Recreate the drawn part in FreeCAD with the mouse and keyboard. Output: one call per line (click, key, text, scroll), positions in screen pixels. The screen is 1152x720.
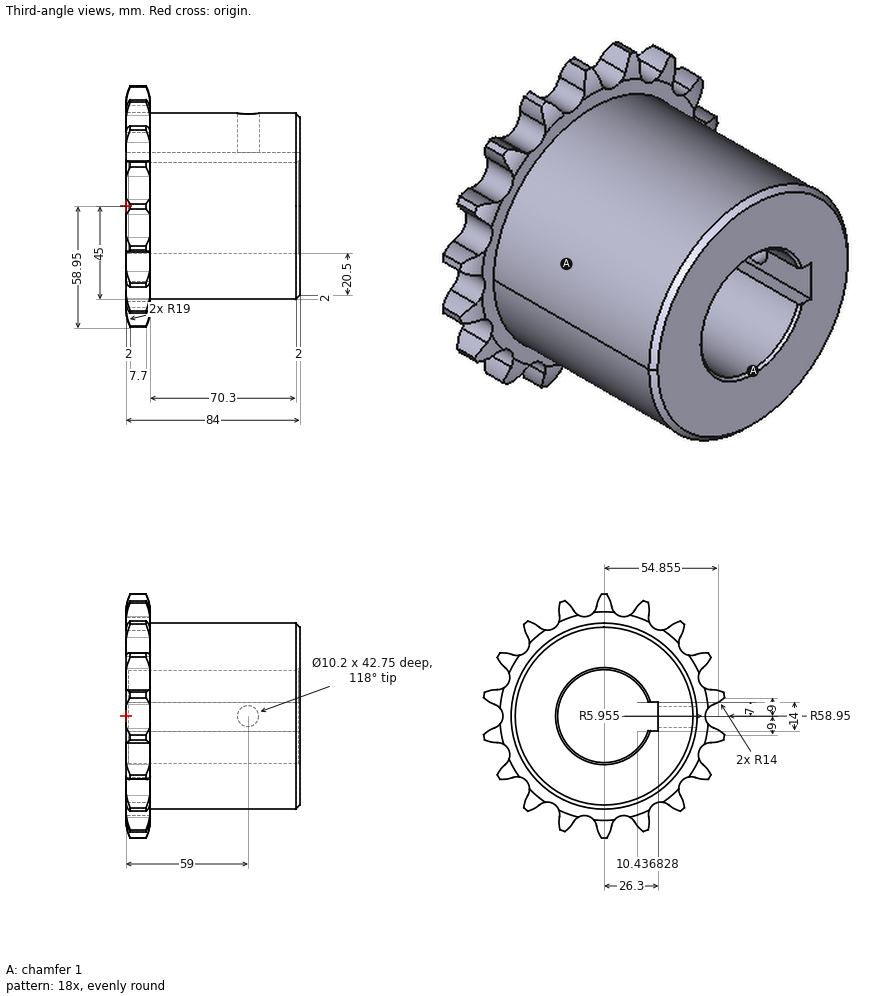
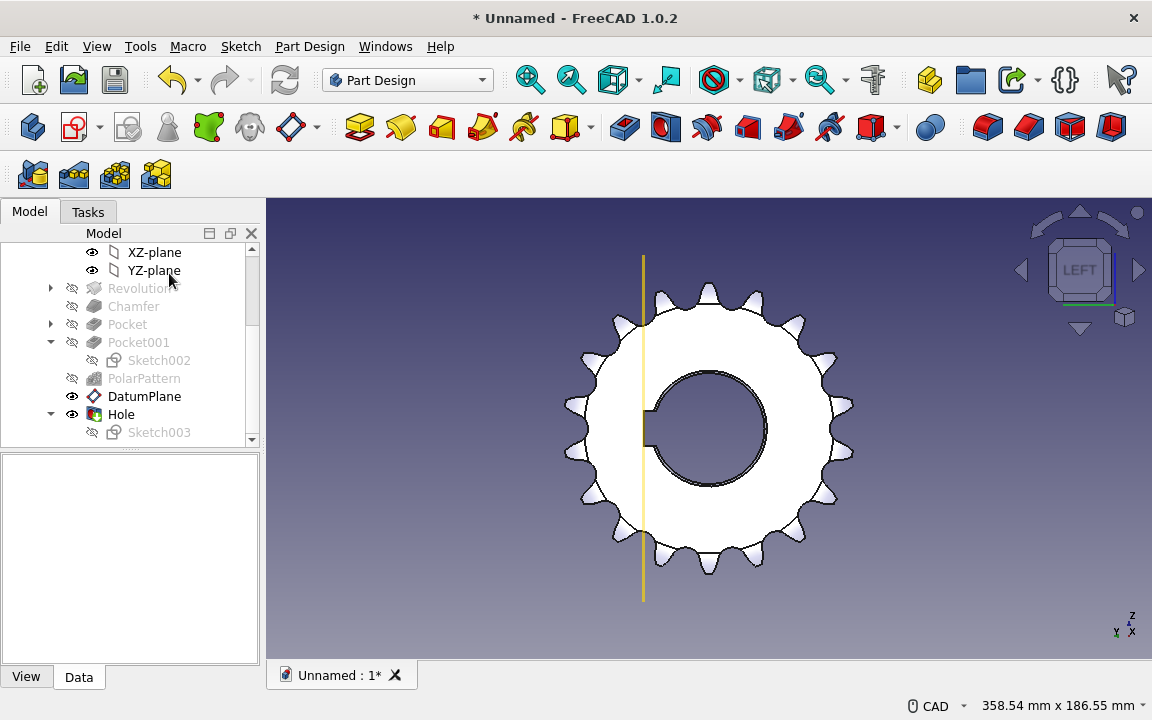
click(117, 396)
key(space)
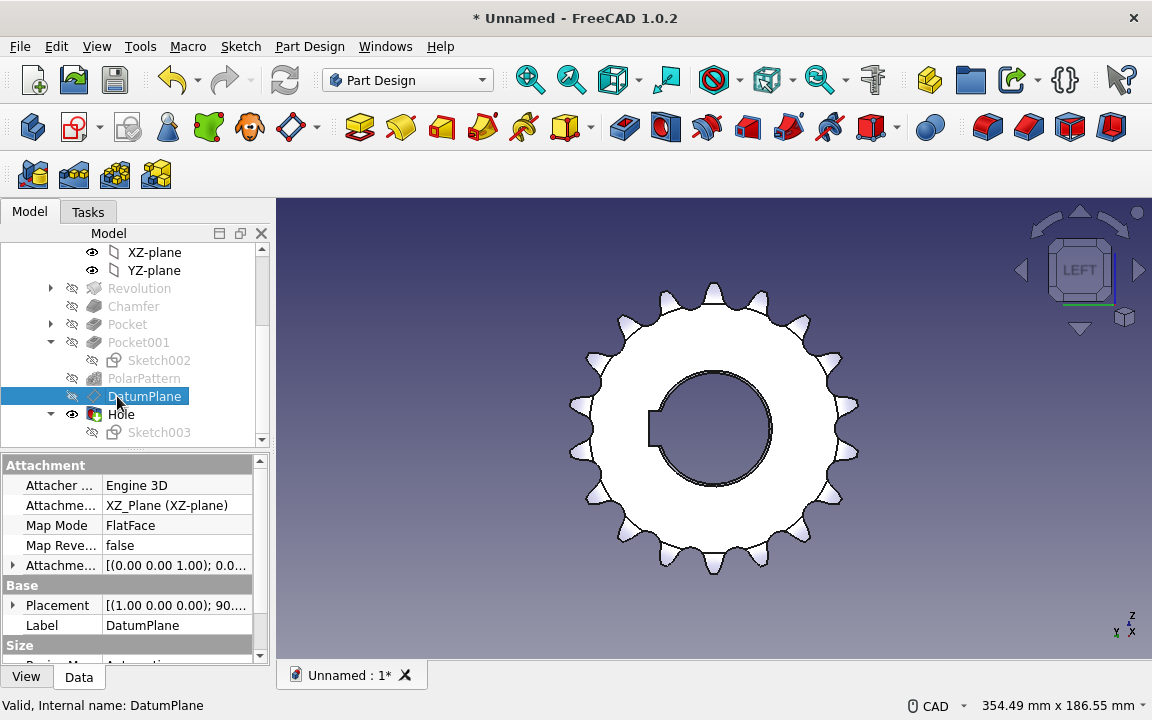
key(0)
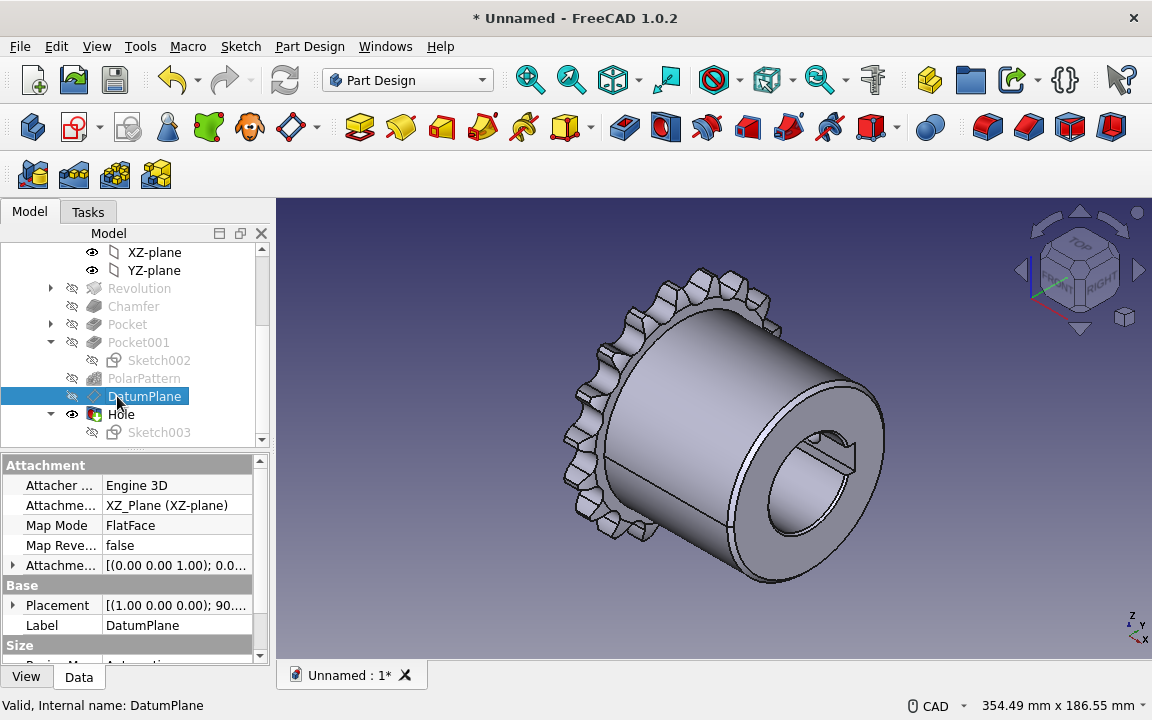
click(531, 80)